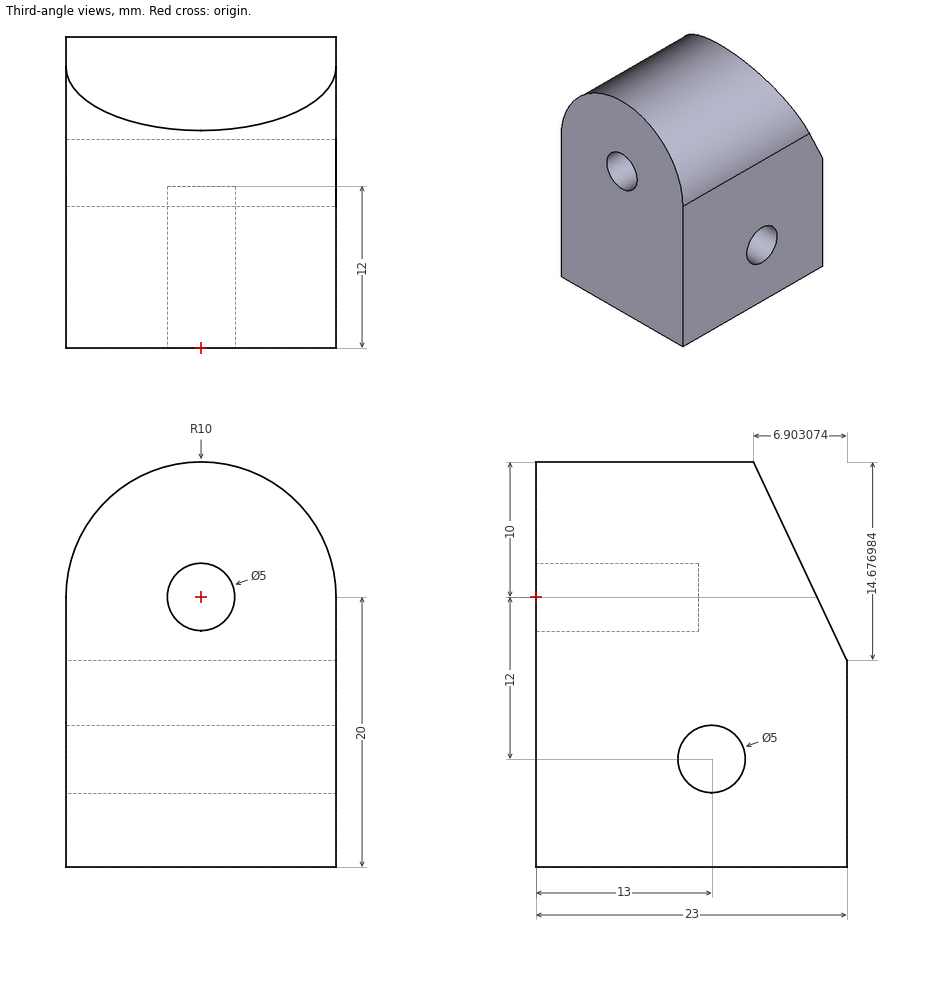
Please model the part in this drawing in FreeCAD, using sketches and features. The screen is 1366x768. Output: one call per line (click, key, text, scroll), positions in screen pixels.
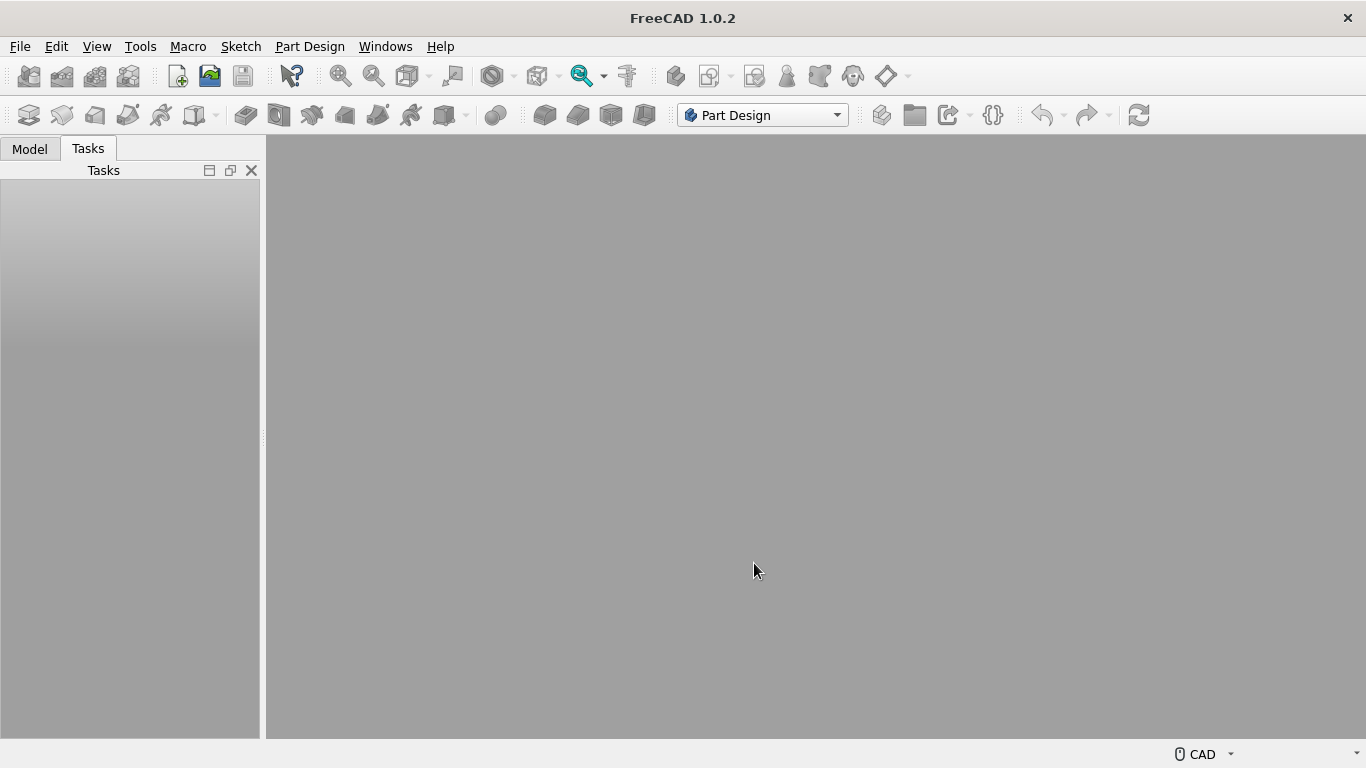
click(177, 76)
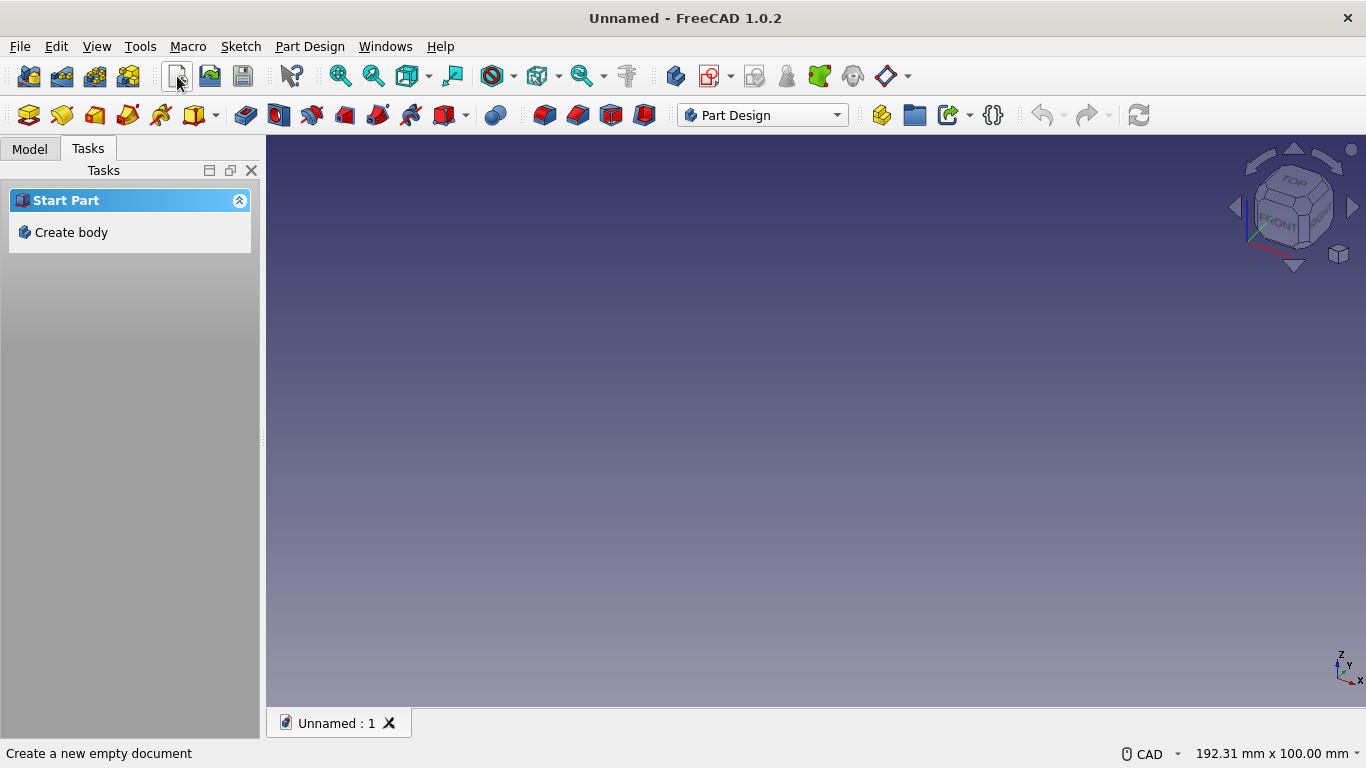
click(708, 76)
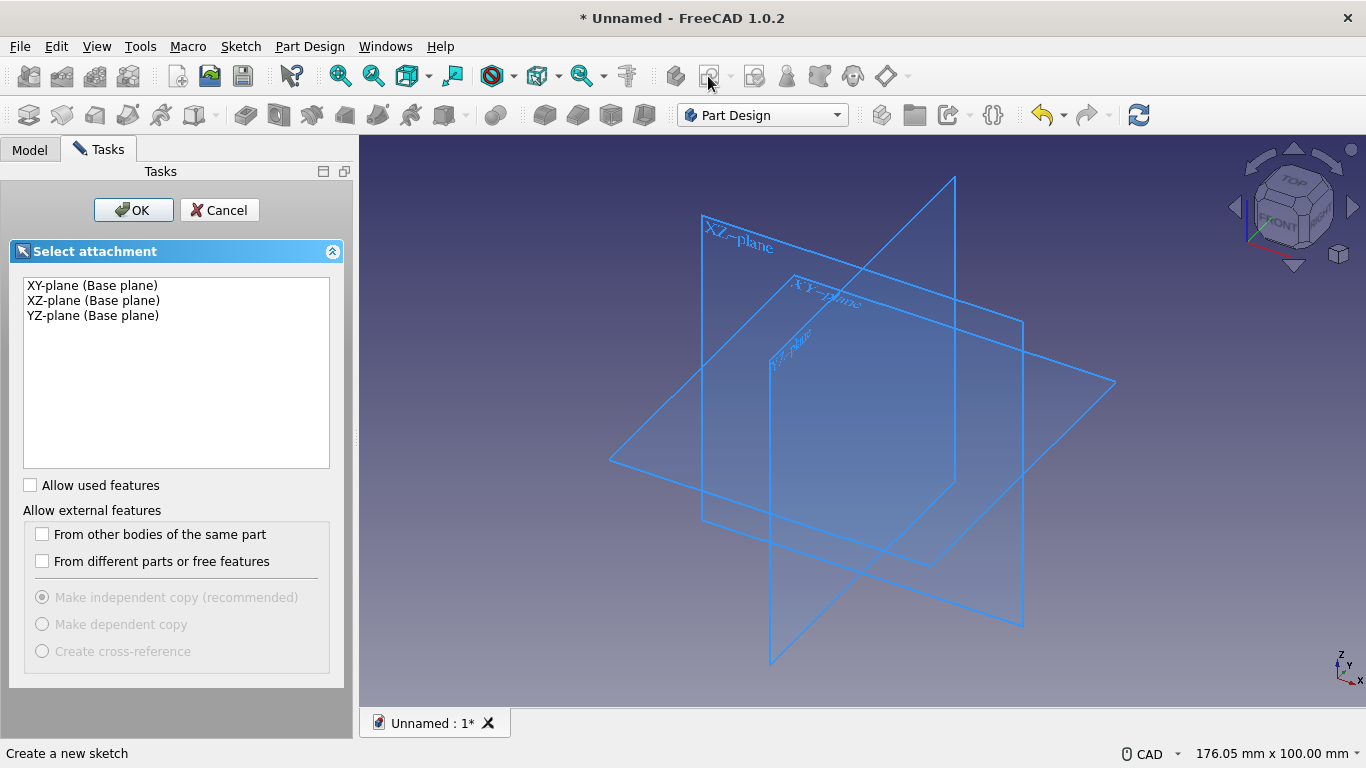
click(84, 300)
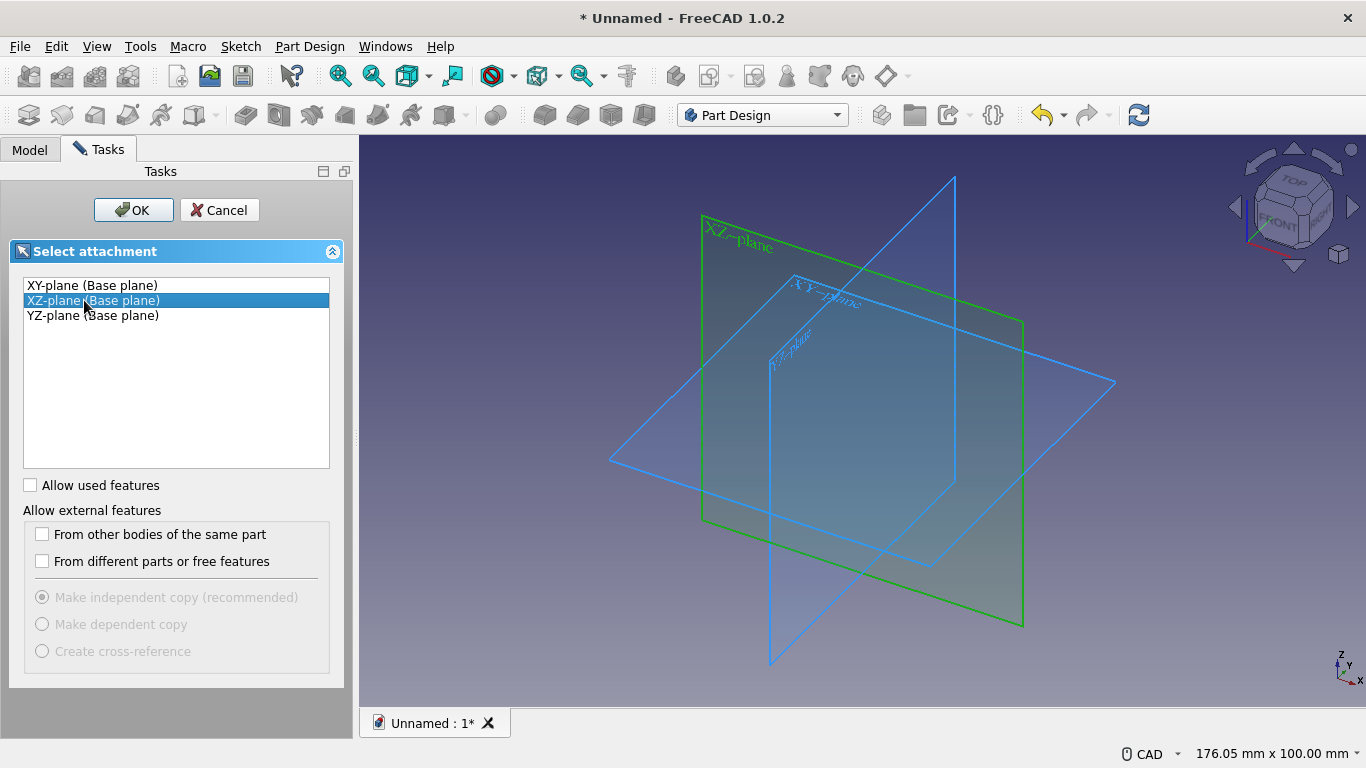
click(134, 210)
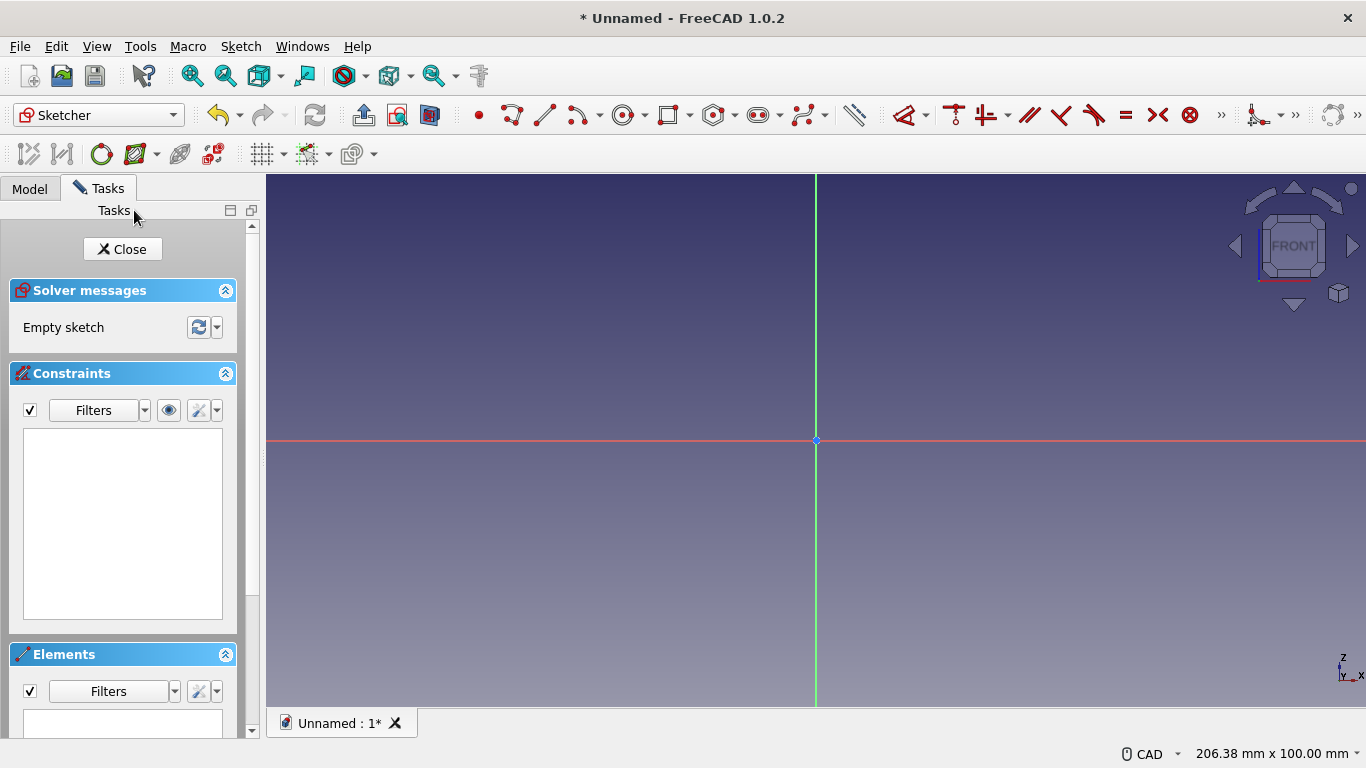
scroll(872, 489, up, 4)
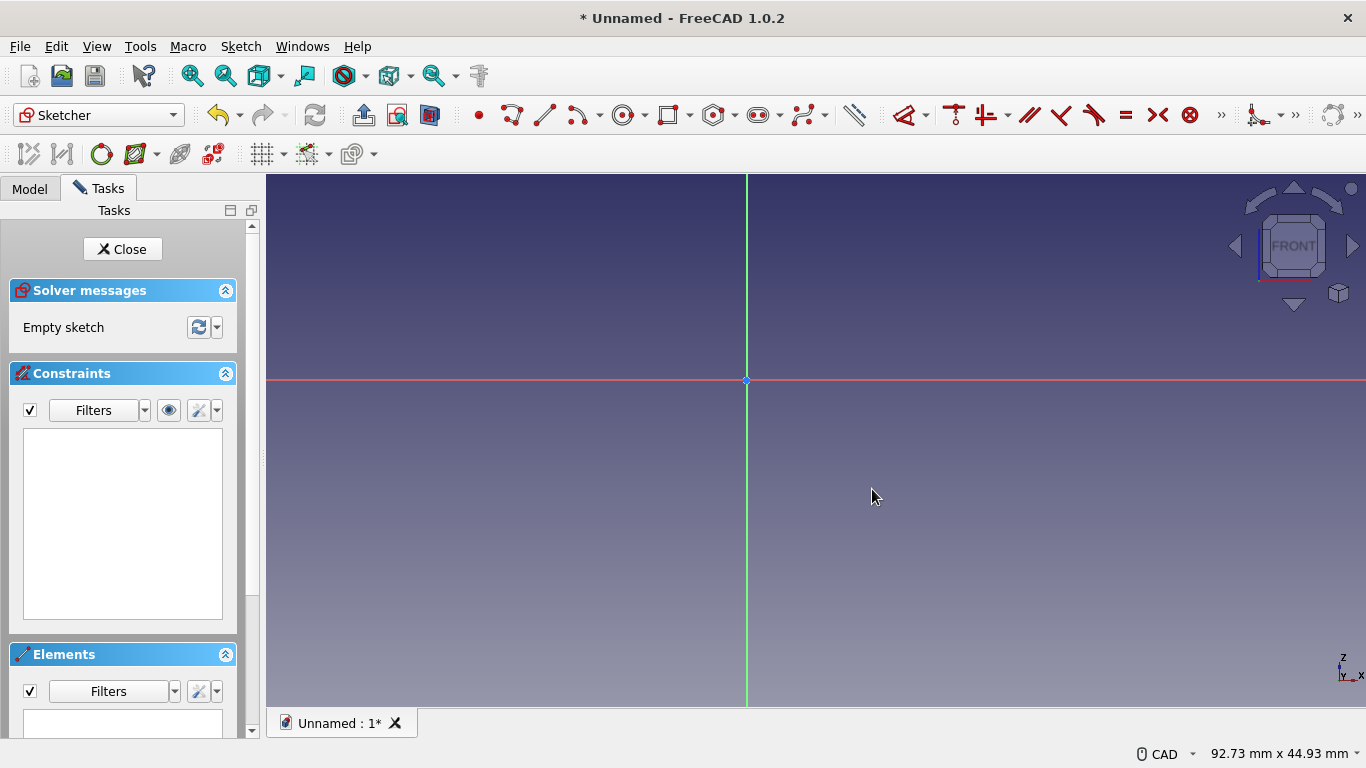
click(512, 116)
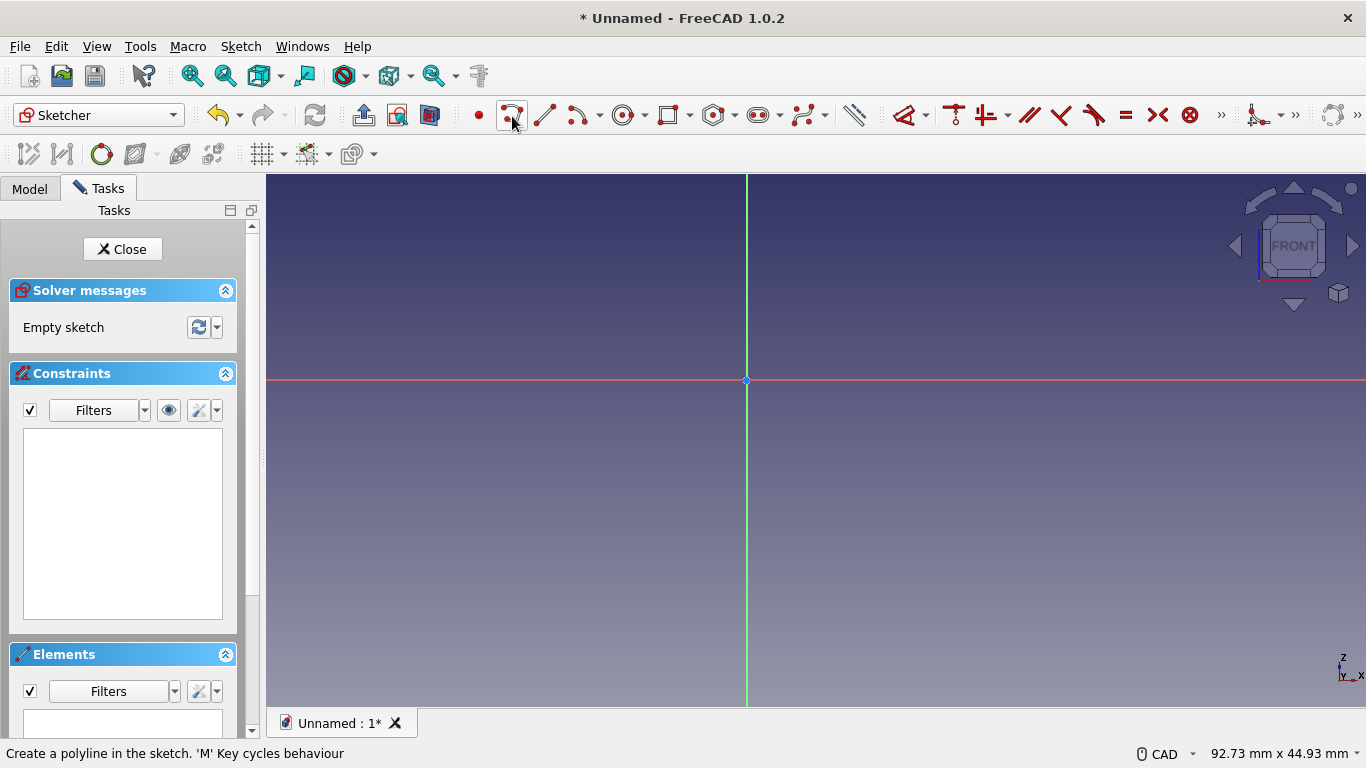
click(865, 380)
click(865, 618)
click(628, 618)
click(628, 380)
right_click(628, 380)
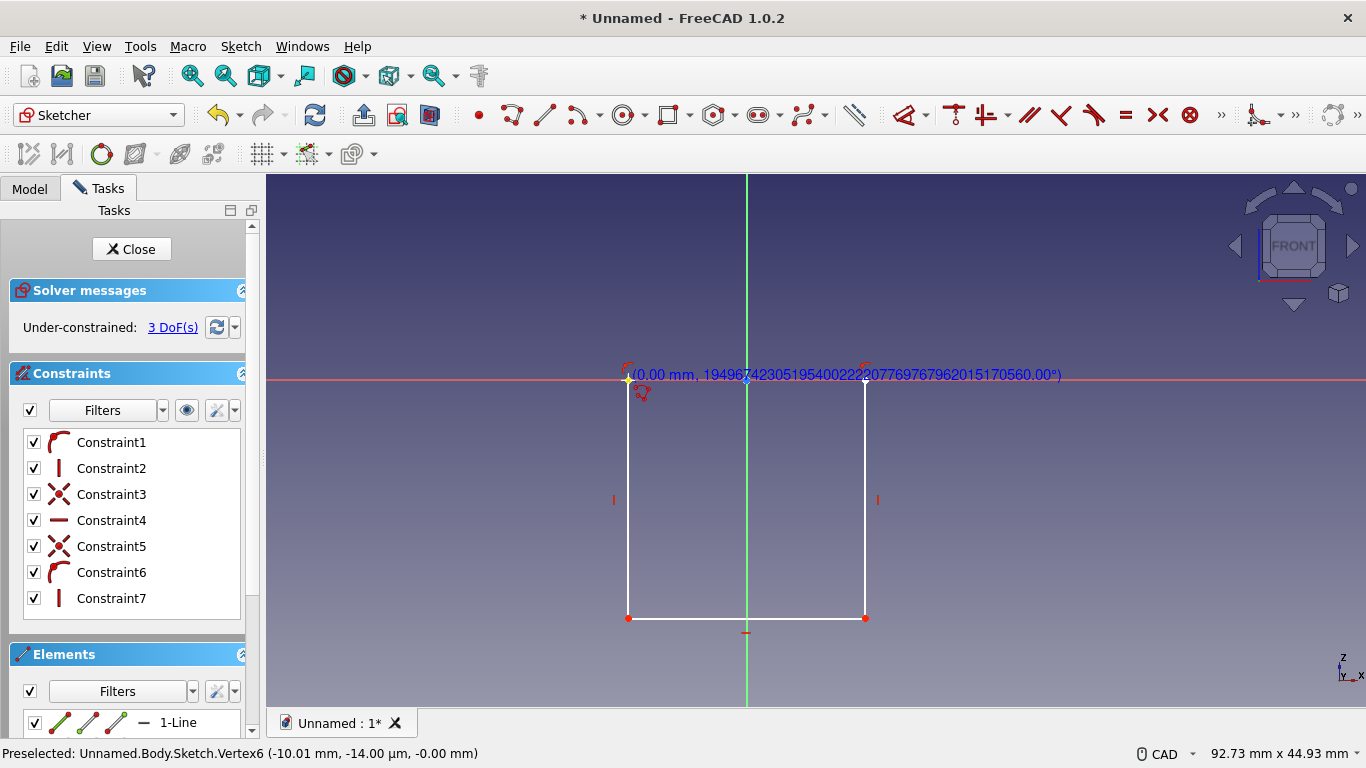
key(g)
key(3)
key(a)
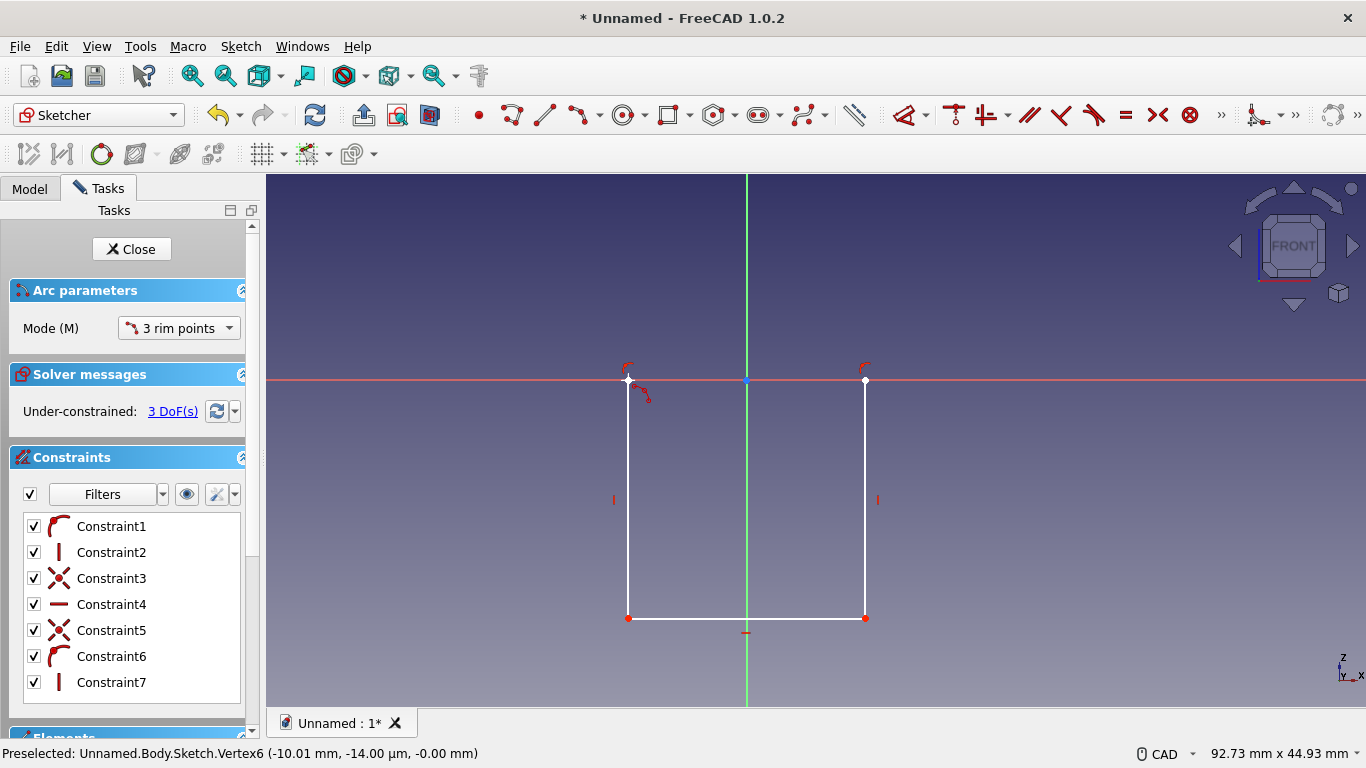
click(628, 380)
click(865, 380)
click(783, 268)
key(Escape)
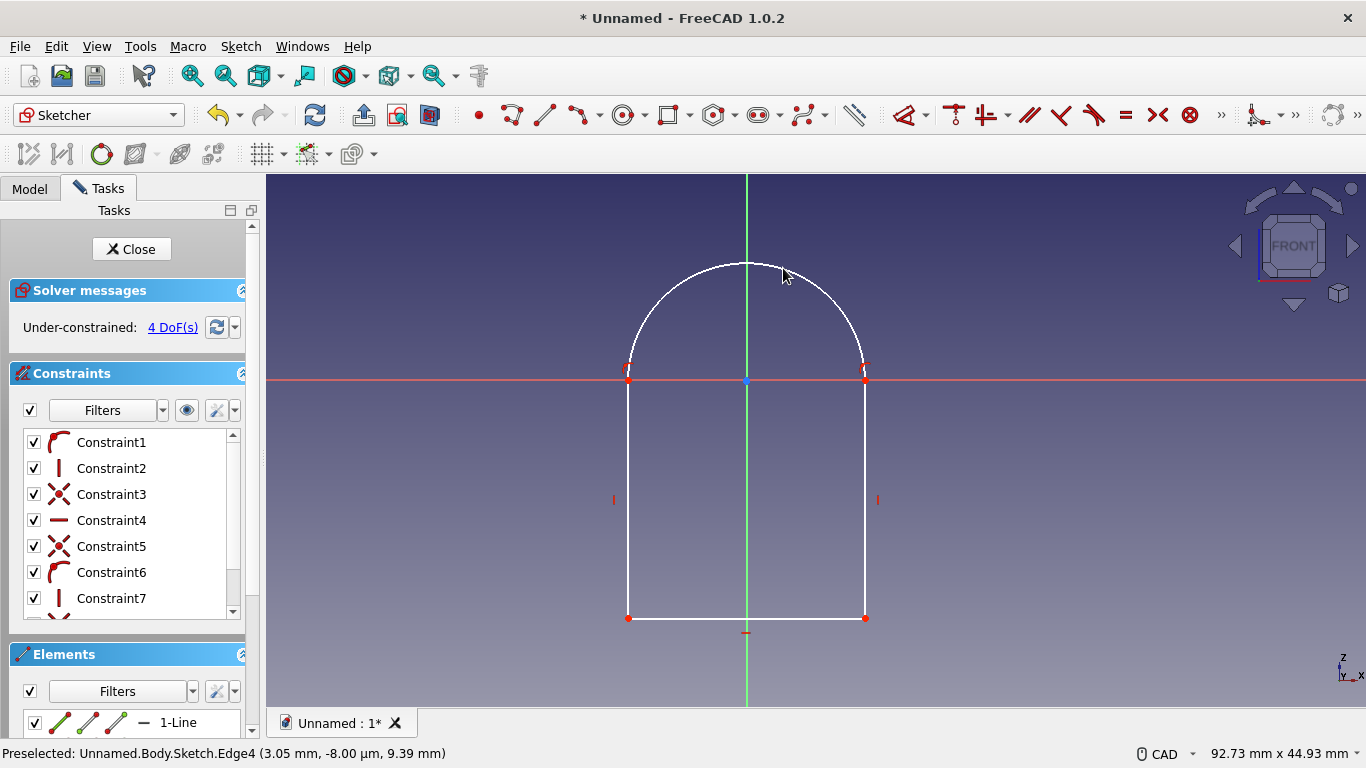
click(865, 452)